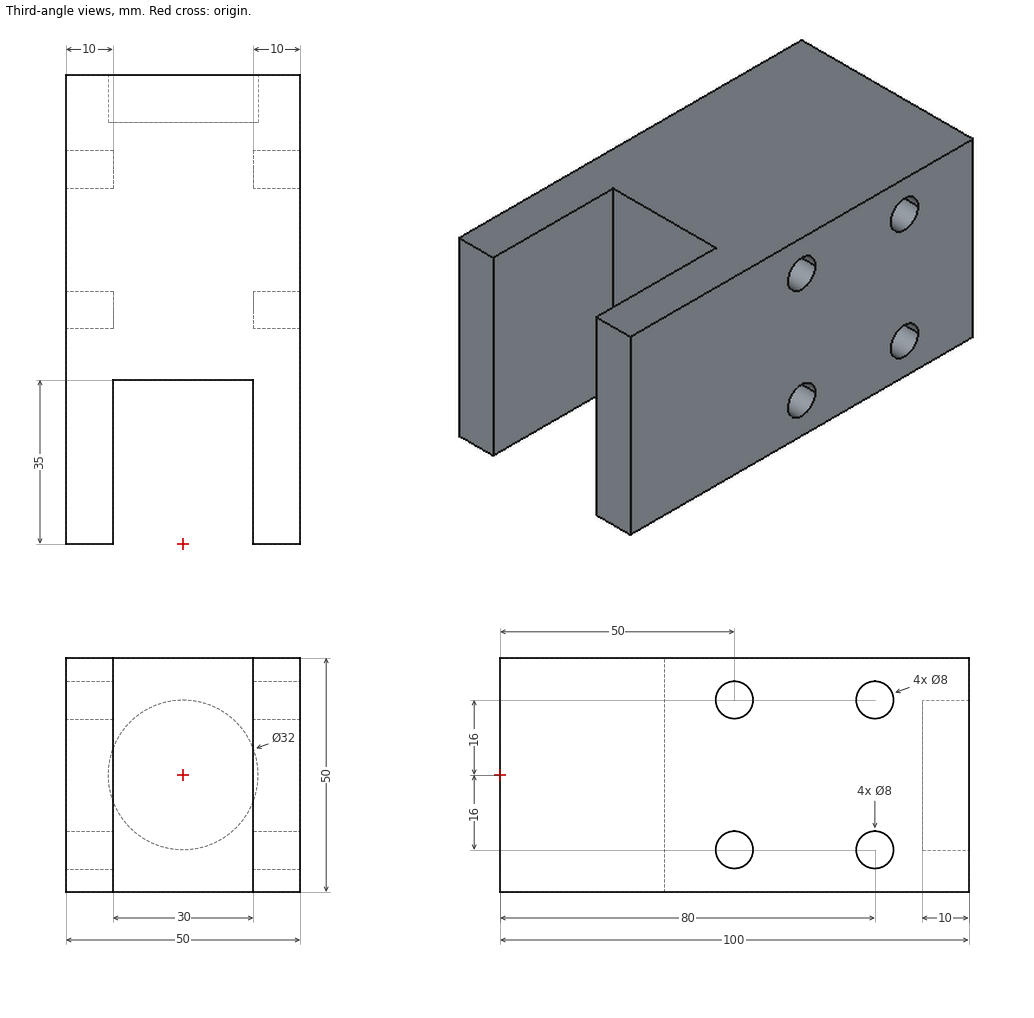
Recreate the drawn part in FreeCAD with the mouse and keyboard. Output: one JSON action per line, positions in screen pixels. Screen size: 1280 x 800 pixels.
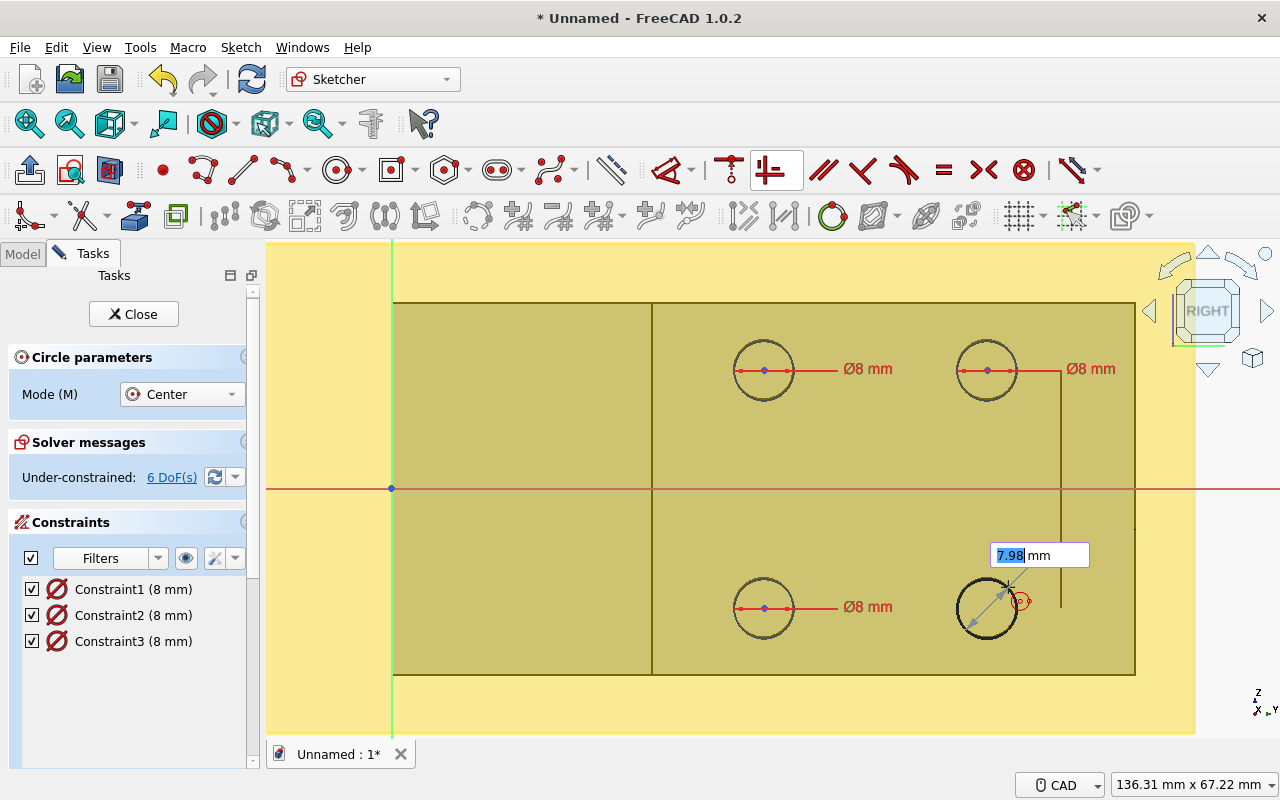
{"action": "type", "text": "8"}
{"action": "key", "text": "Return"}
{"action": "key", "text": "Escape"}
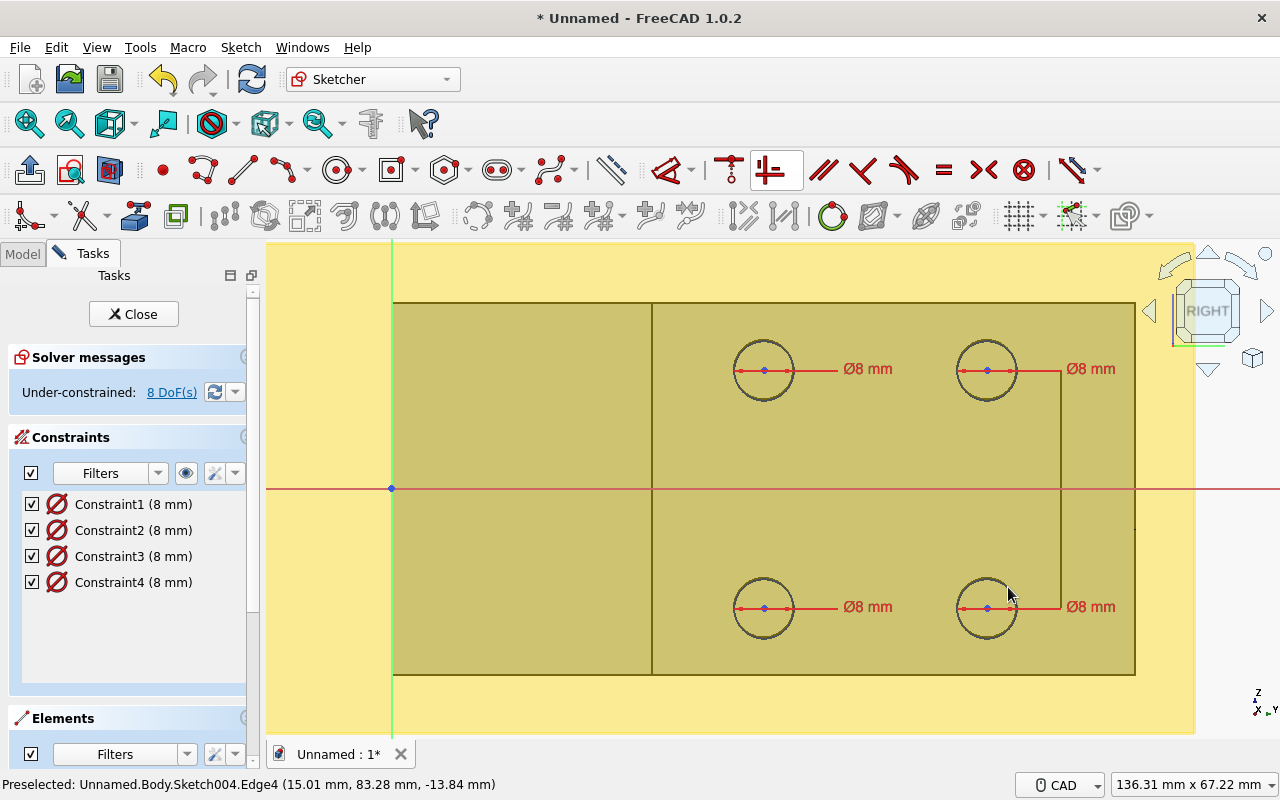
{"action": "left_click", "coordinate": [987, 371]}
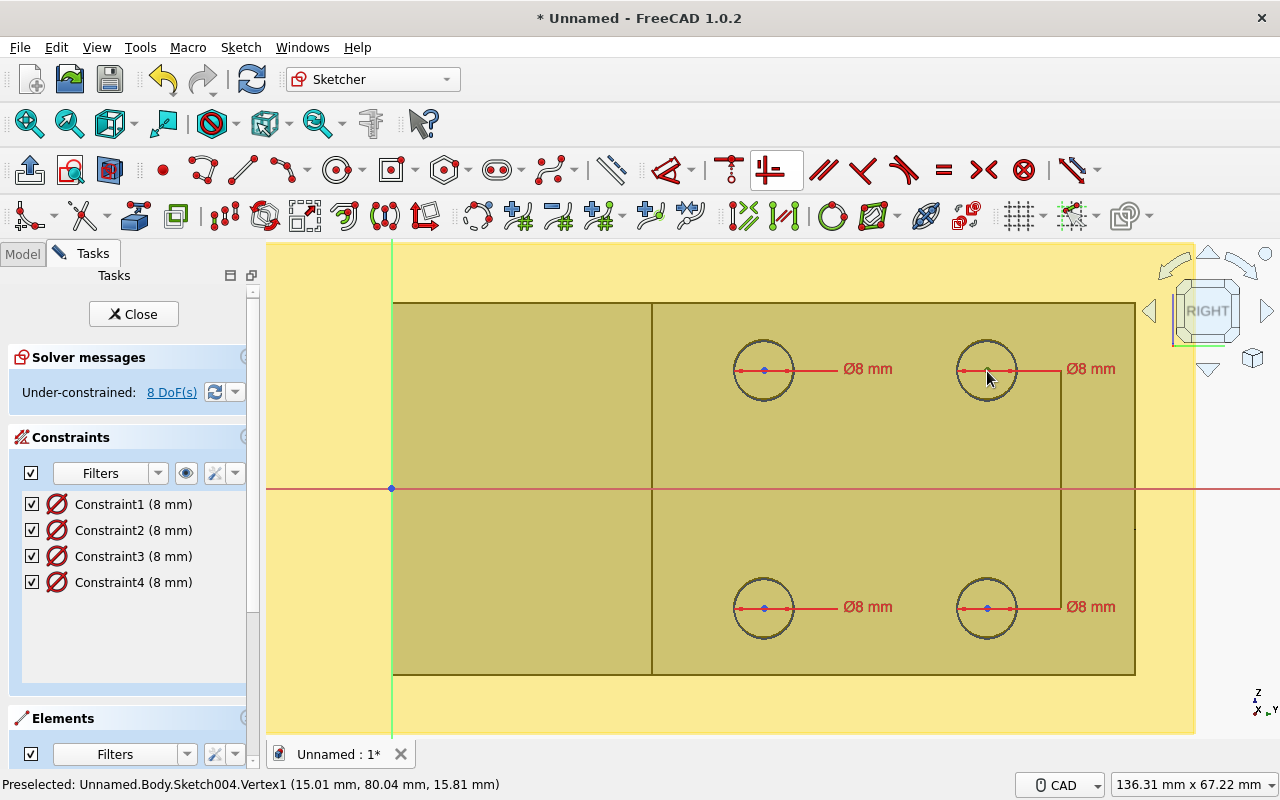
{"action": "left_click", "coordinate": [764, 371]}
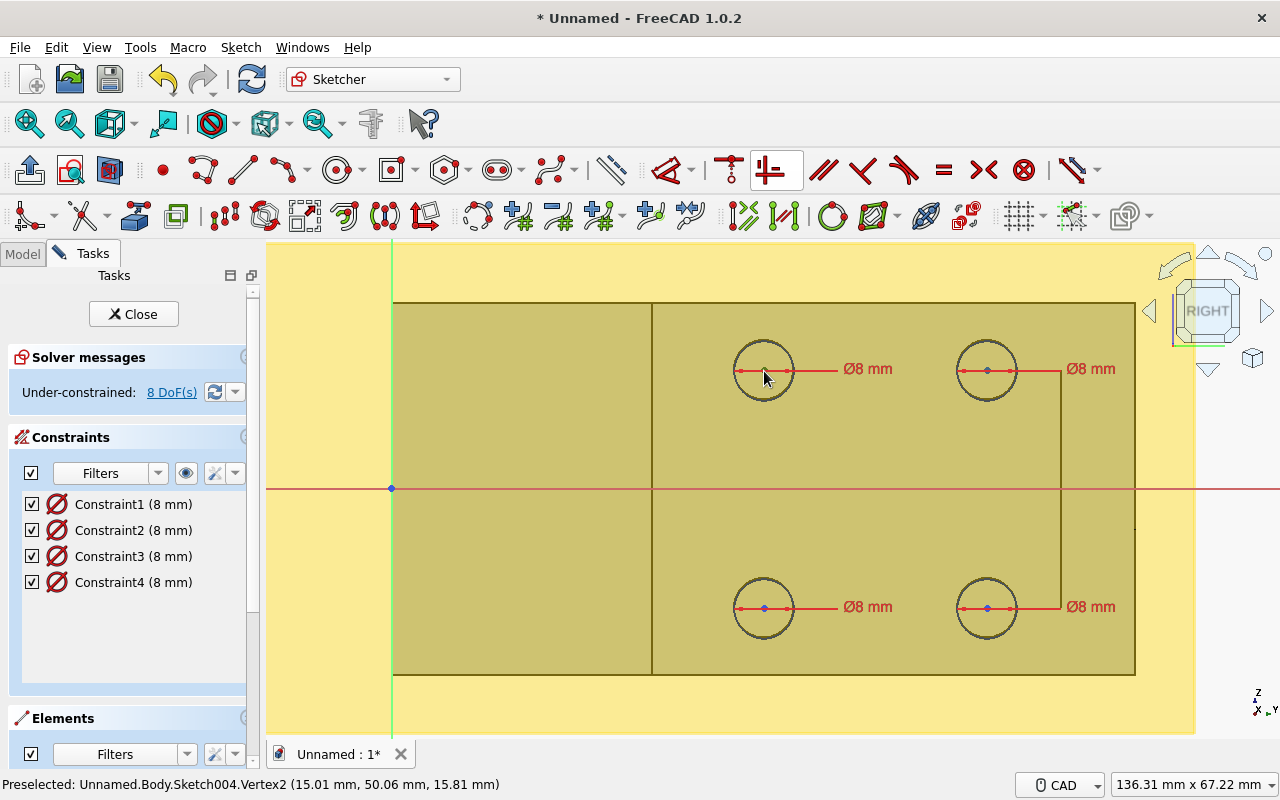
{"action": "key", "text": "h"}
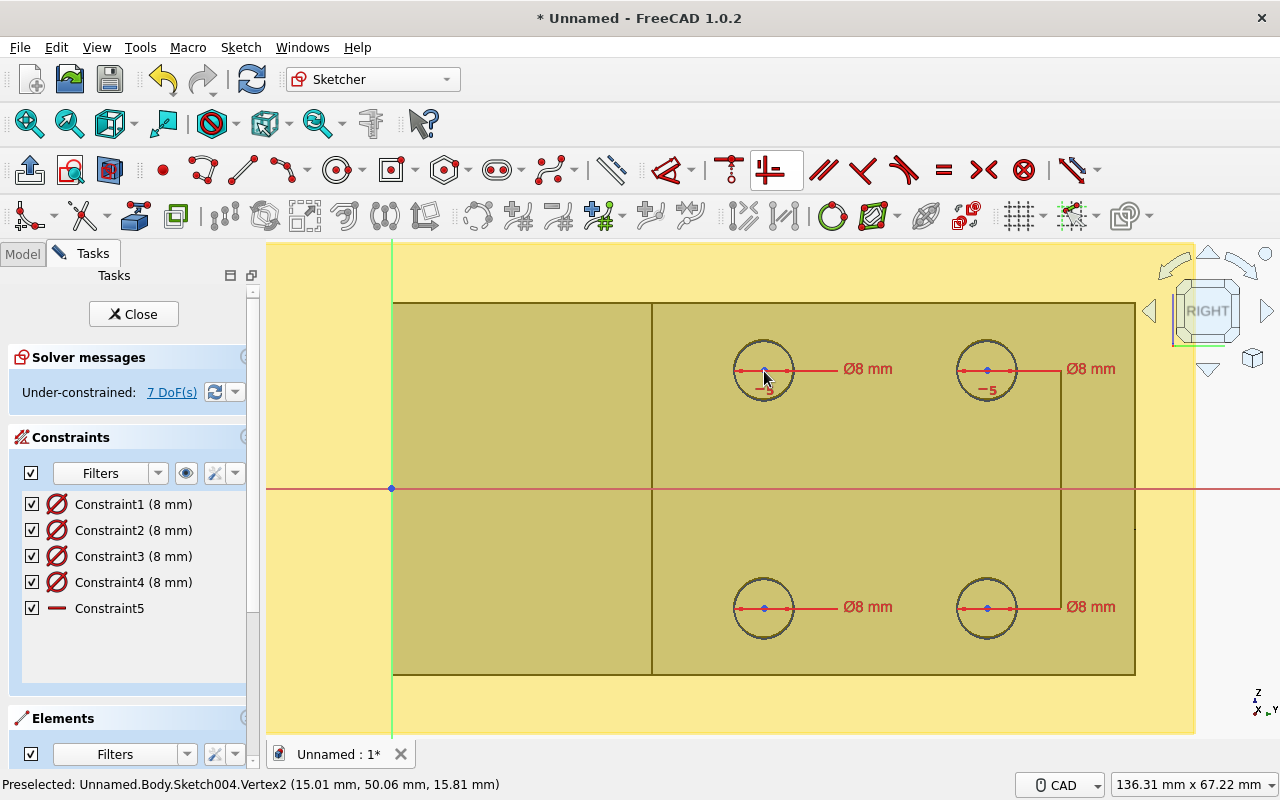
{"action": "left_click", "coordinate": [764, 371]}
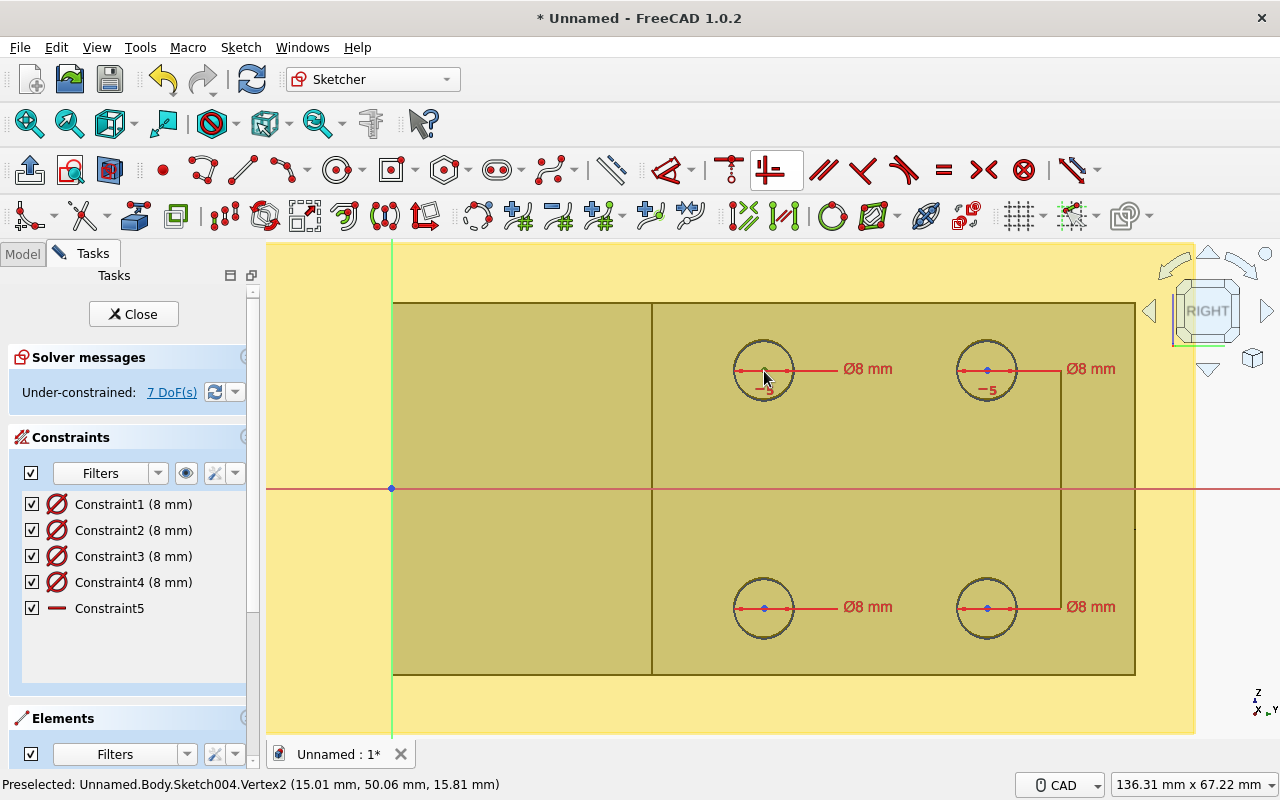
{"action": "left_click", "coordinate": [764, 609]}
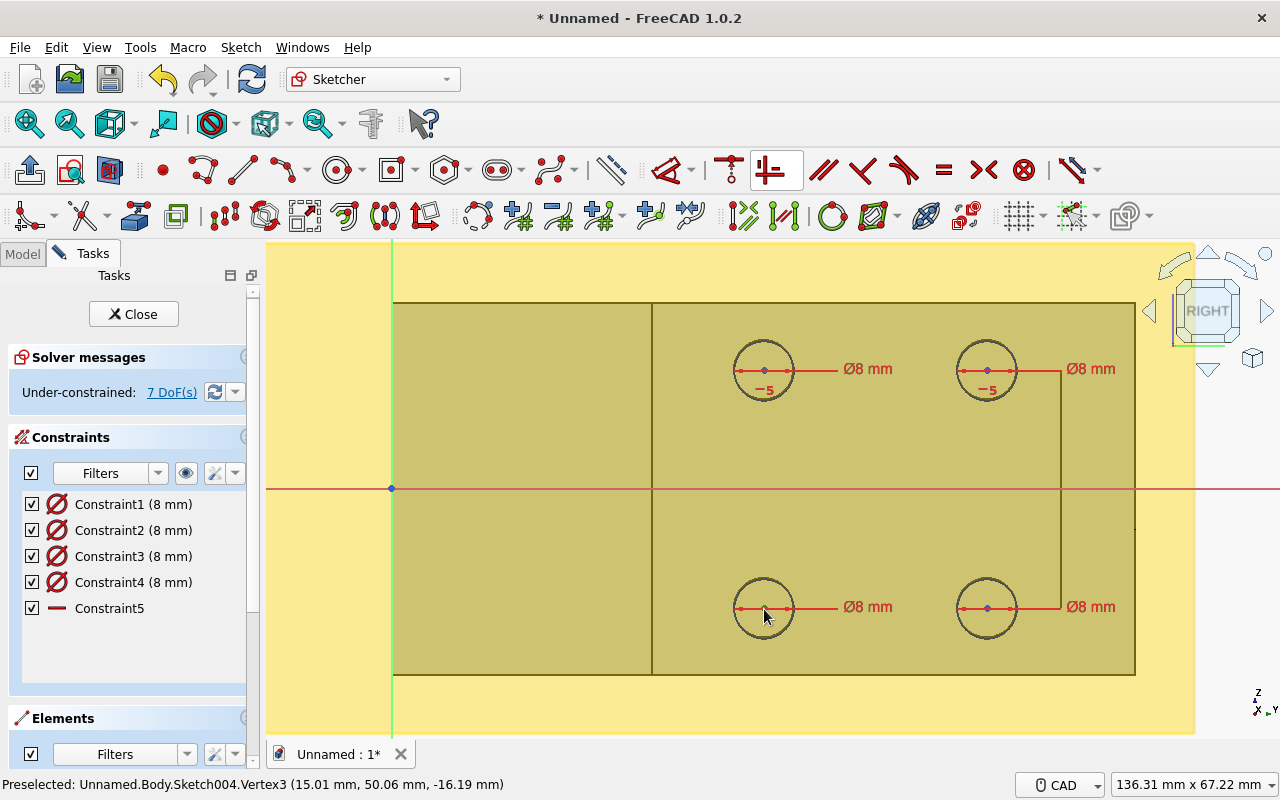
{"action": "key", "text": "v"}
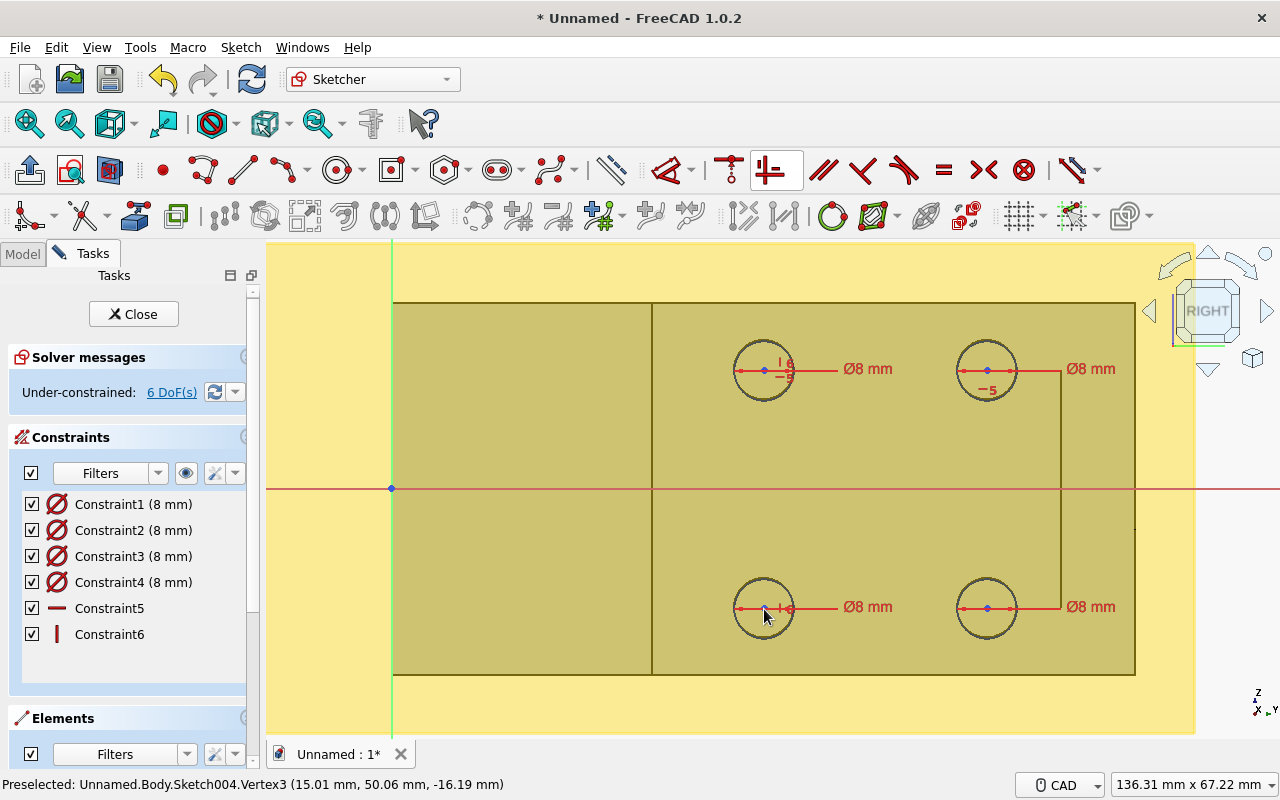
{"action": "left_click", "coordinate": [987, 371]}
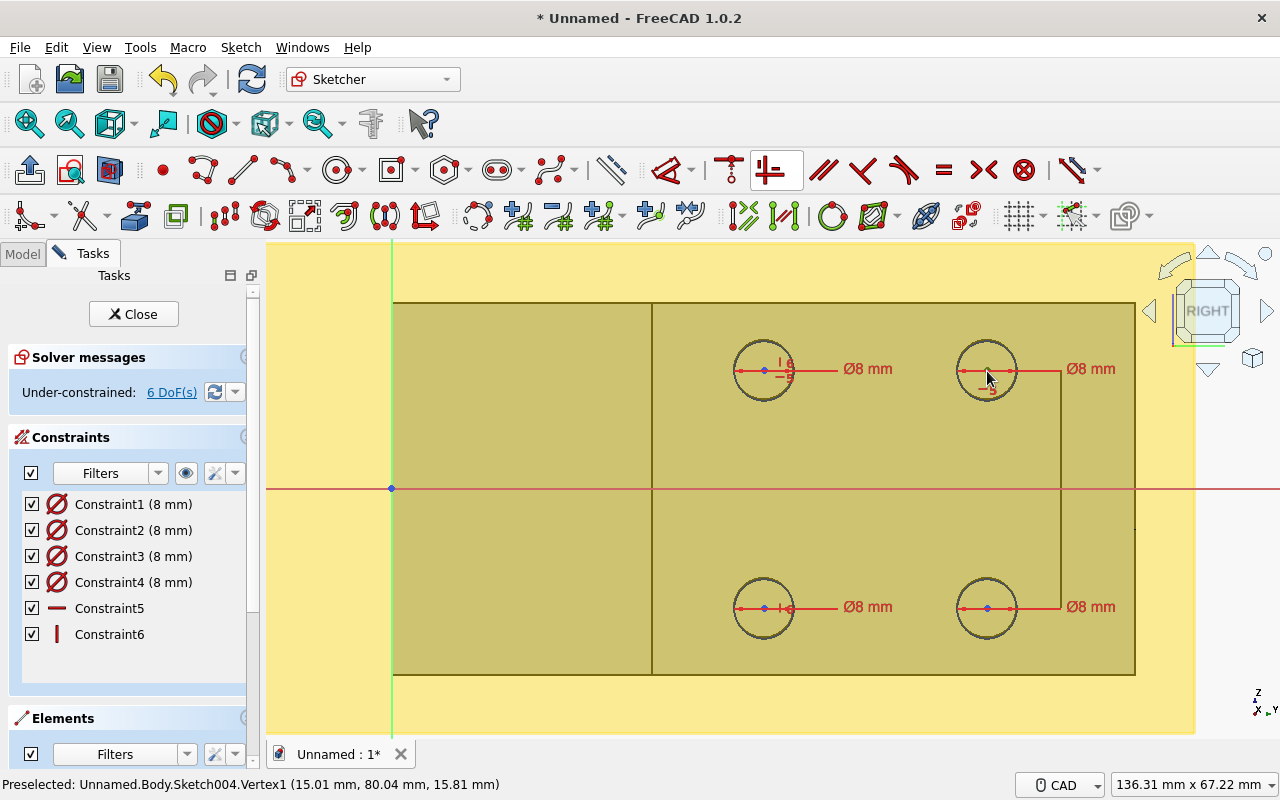
{"action": "left_click", "coordinate": [987, 609]}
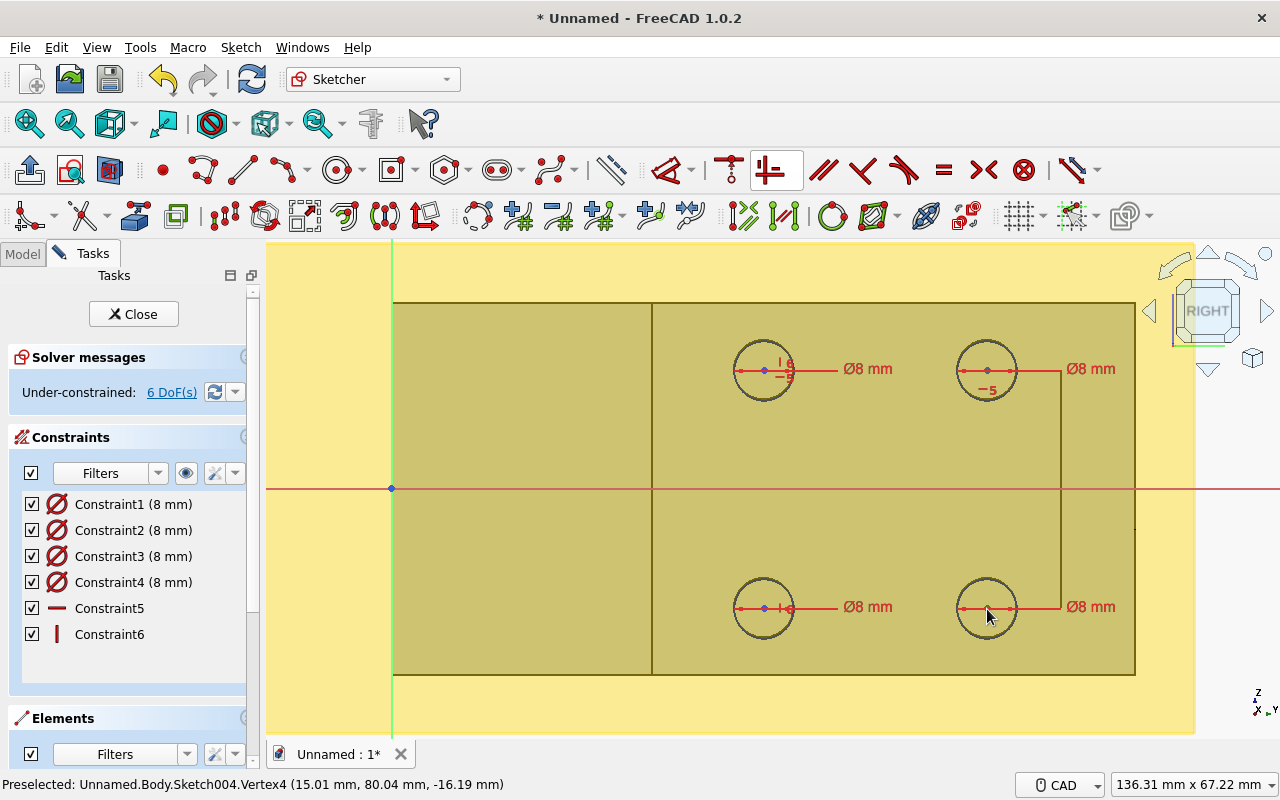
{"action": "left_click", "coordinate": [798, 170]}